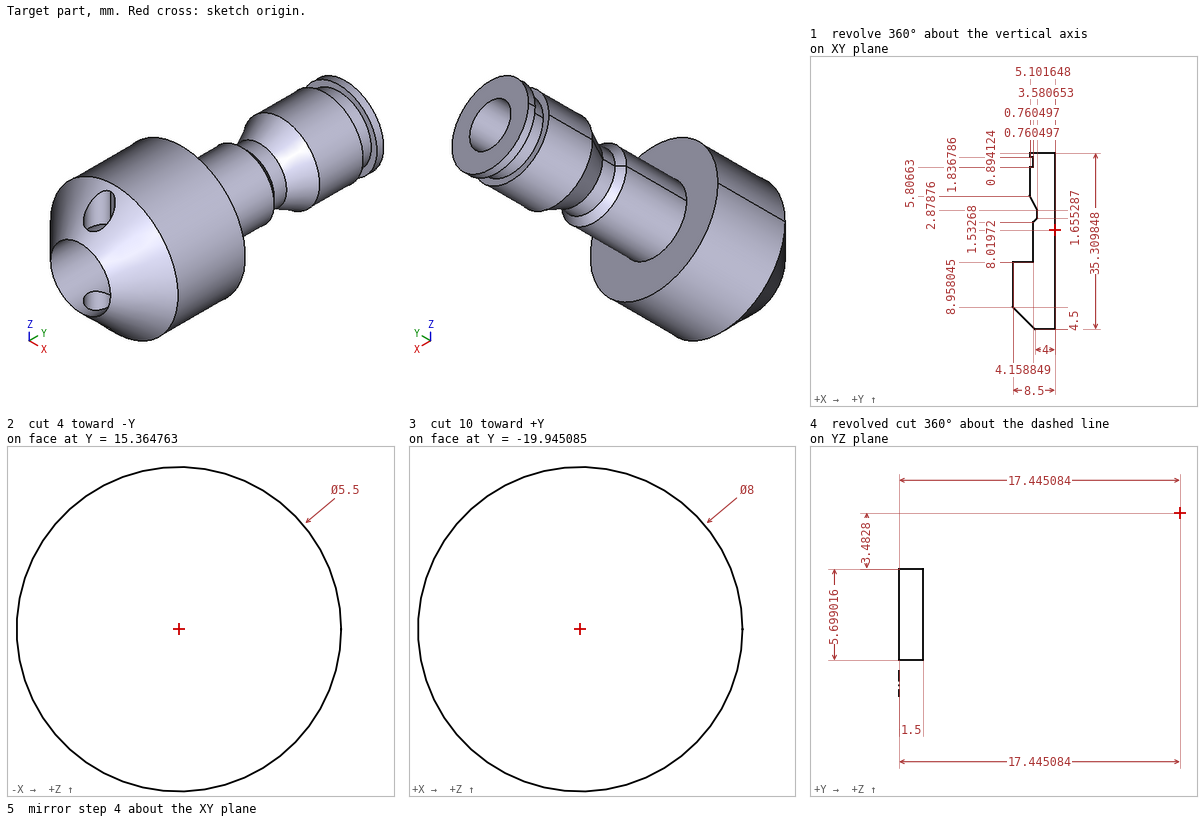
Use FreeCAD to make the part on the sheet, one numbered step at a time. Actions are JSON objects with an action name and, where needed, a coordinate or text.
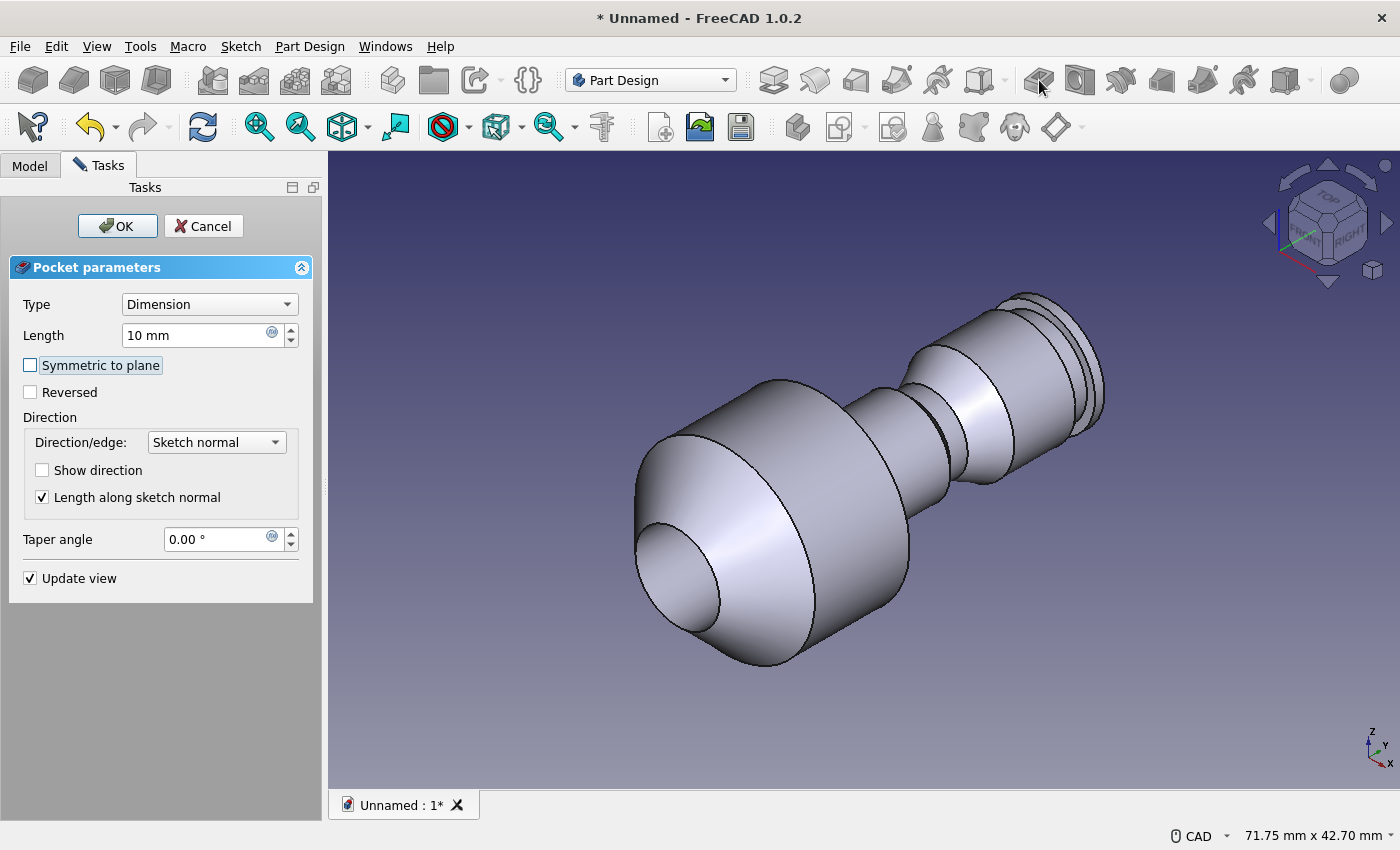
{"action": "left_click", "coordinate": [118, 226]}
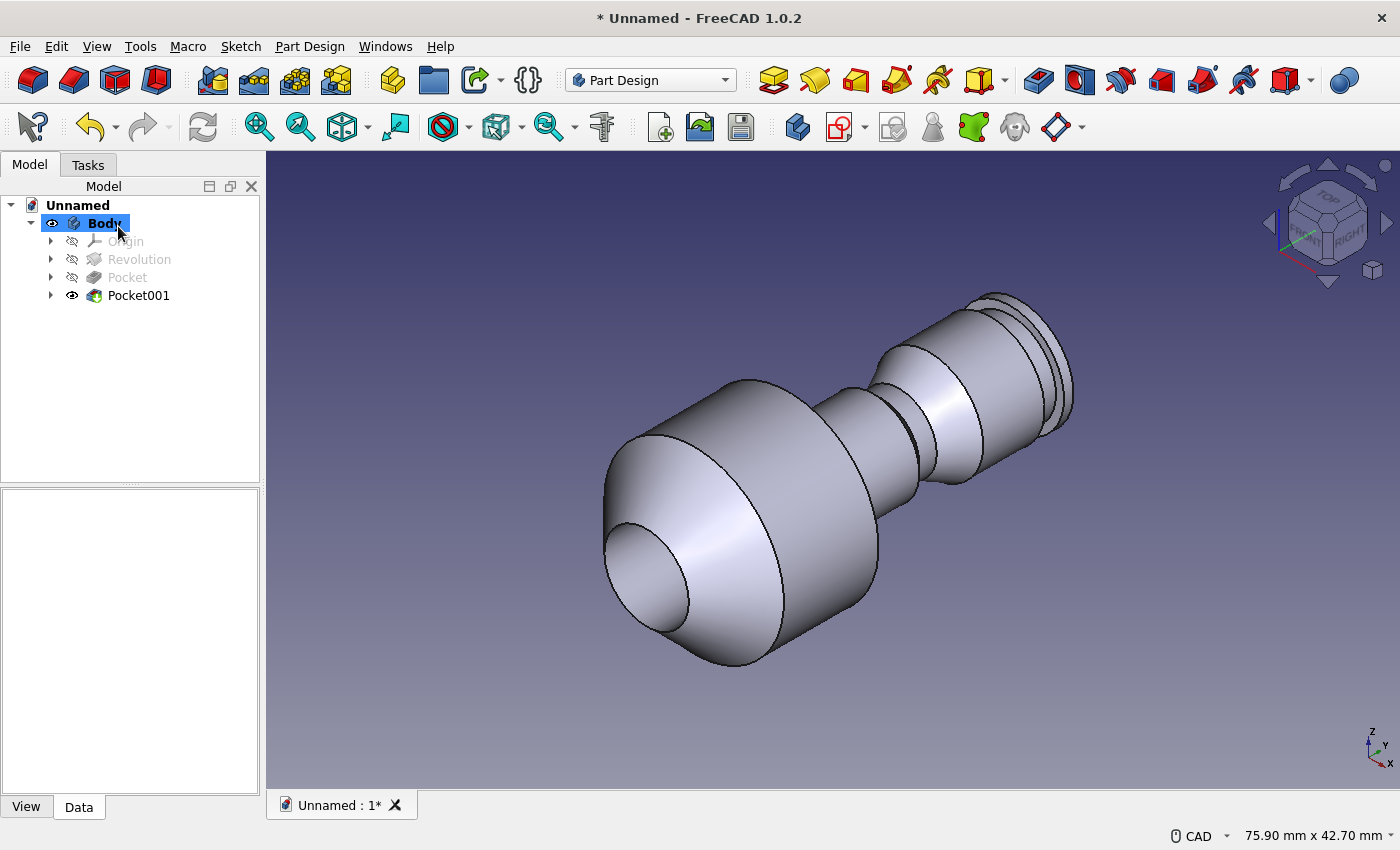
{"action": "left_click", "coordinate": [838, 128]}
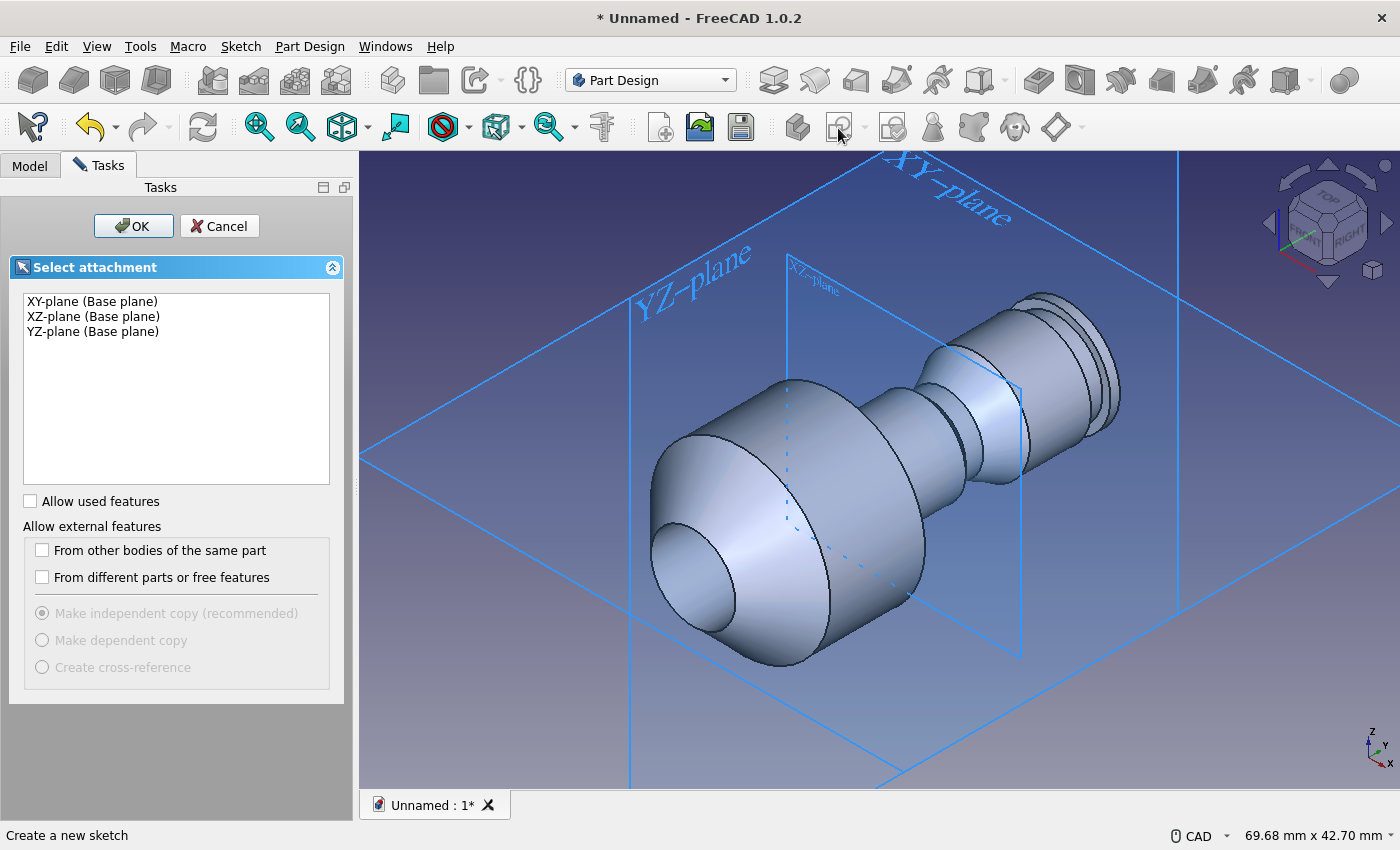
{"action": "left_click", "coordinate": [84, 332]}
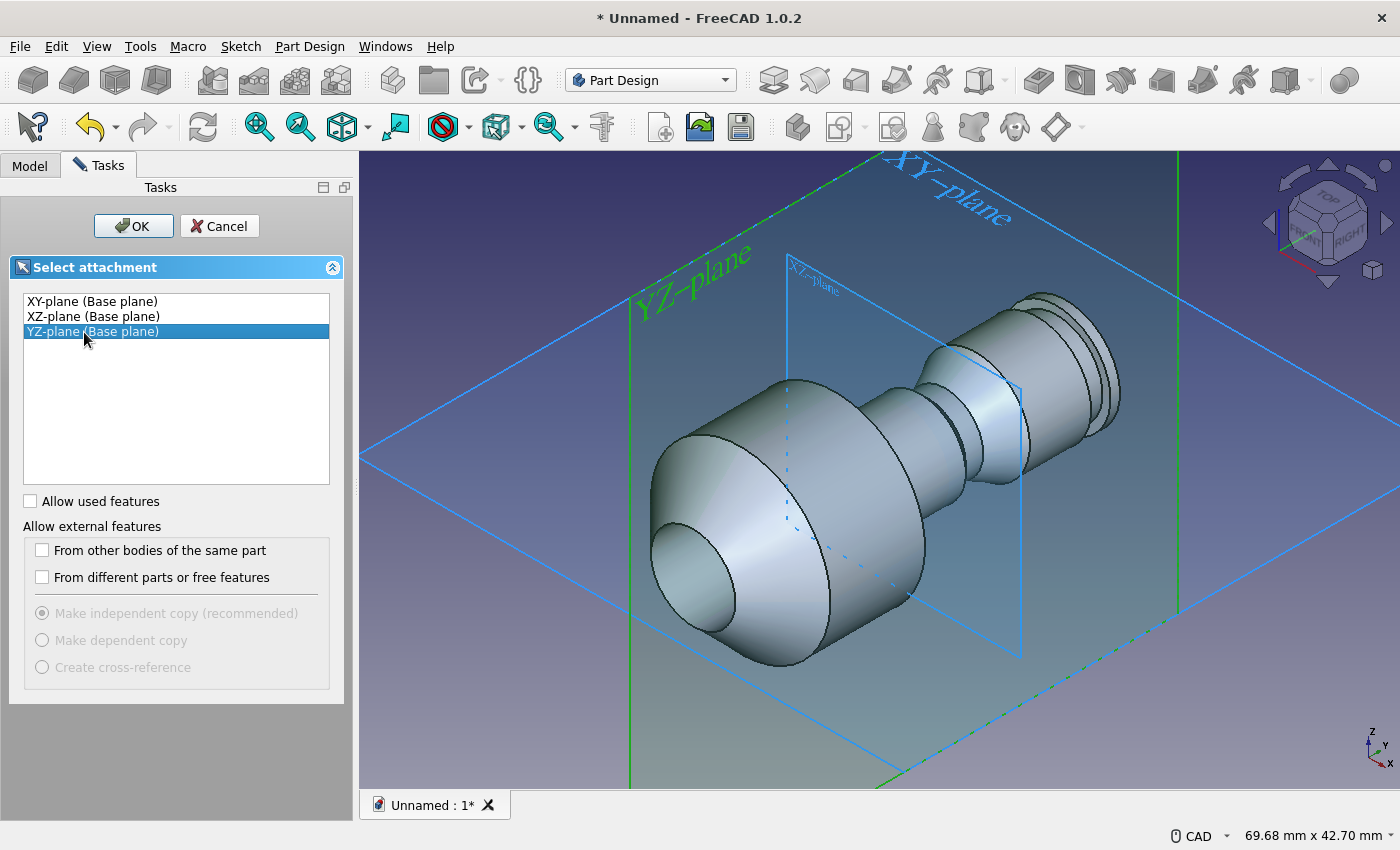
{"action": "left_click", "coordinate": [134, 226]}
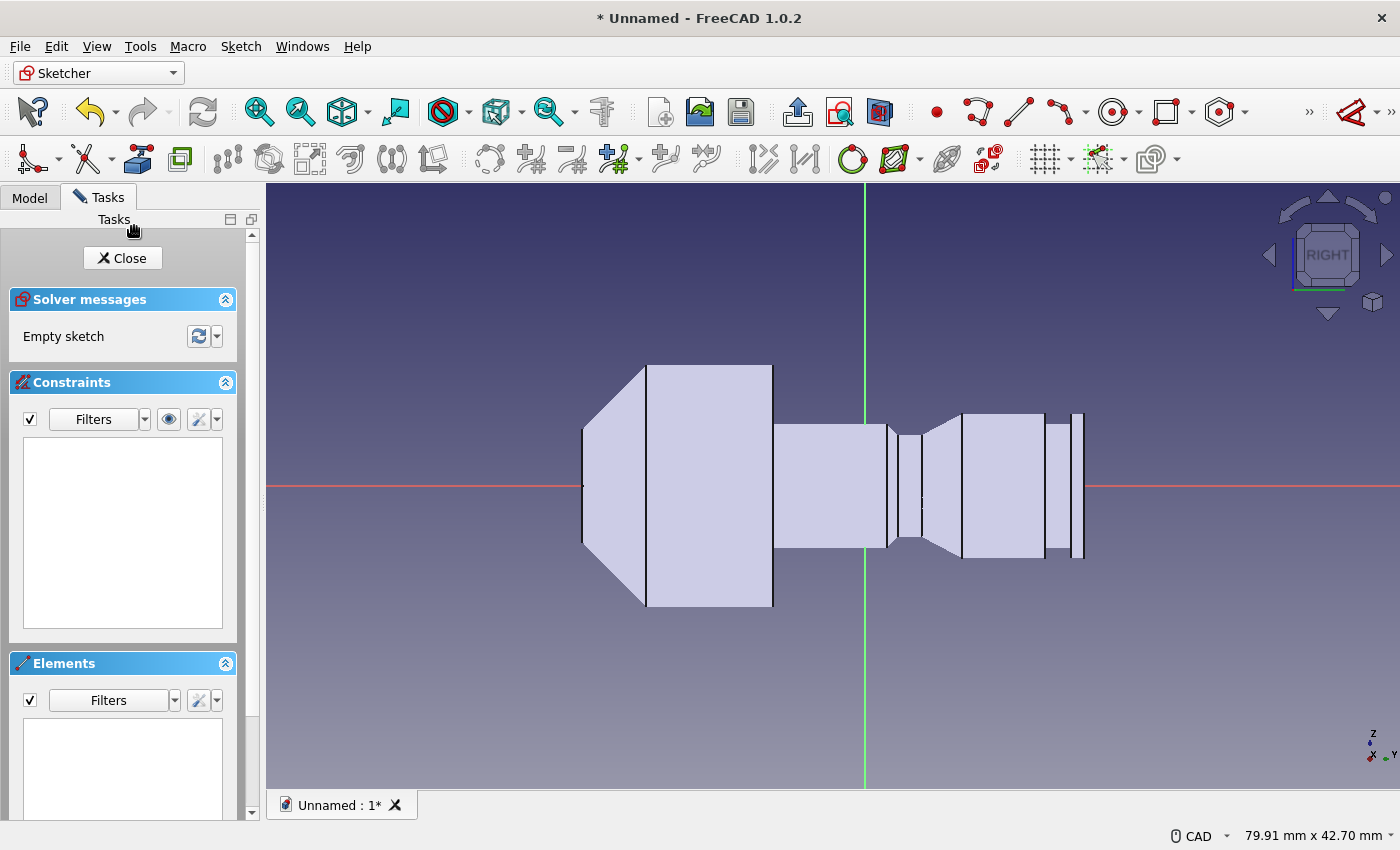
{"action": "left_click", "coordinate": [880, 112]}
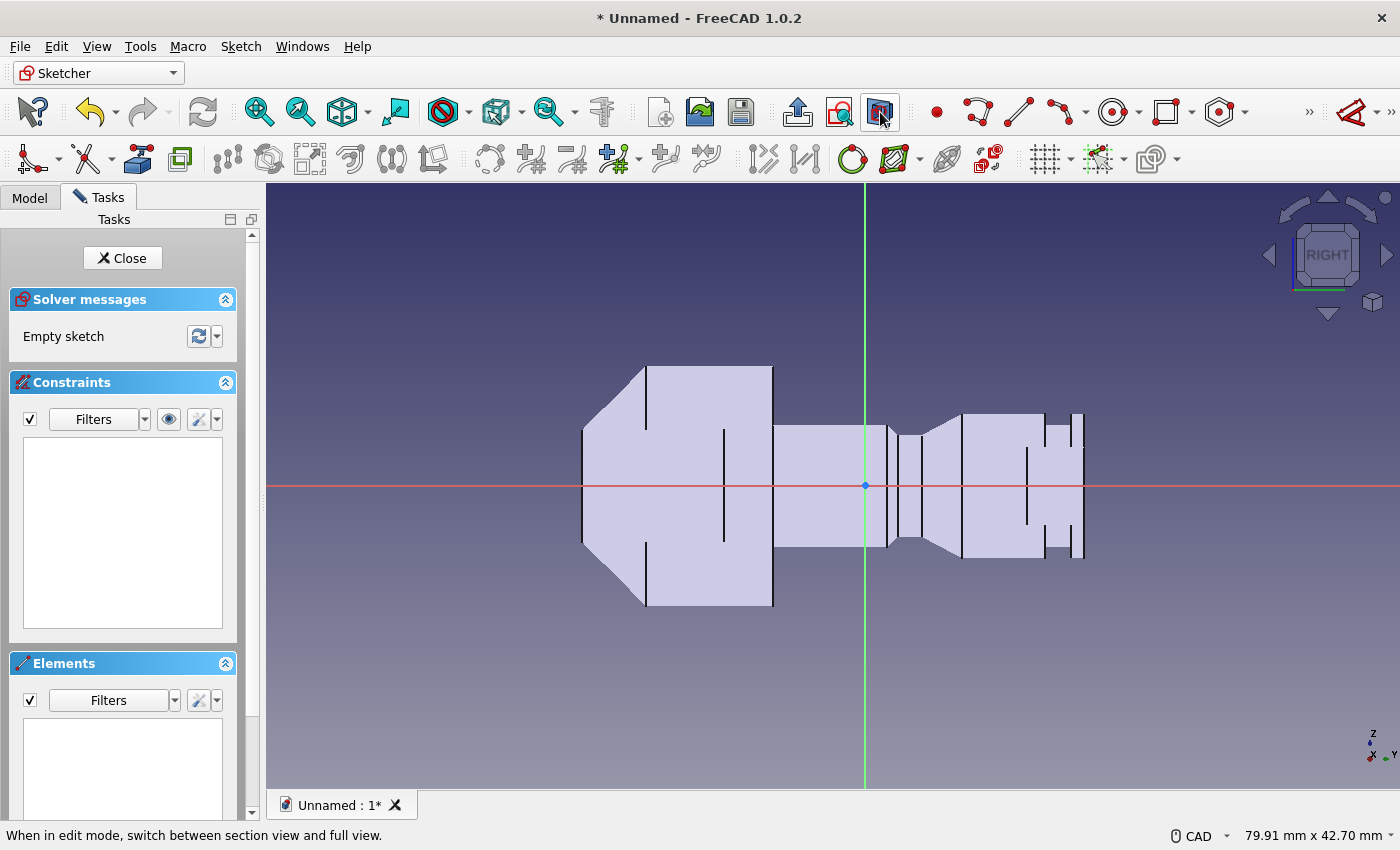
{"action": "scroll", "coordinate": [723, 634], "scroll_direction": "up", "scroll_amount": 4}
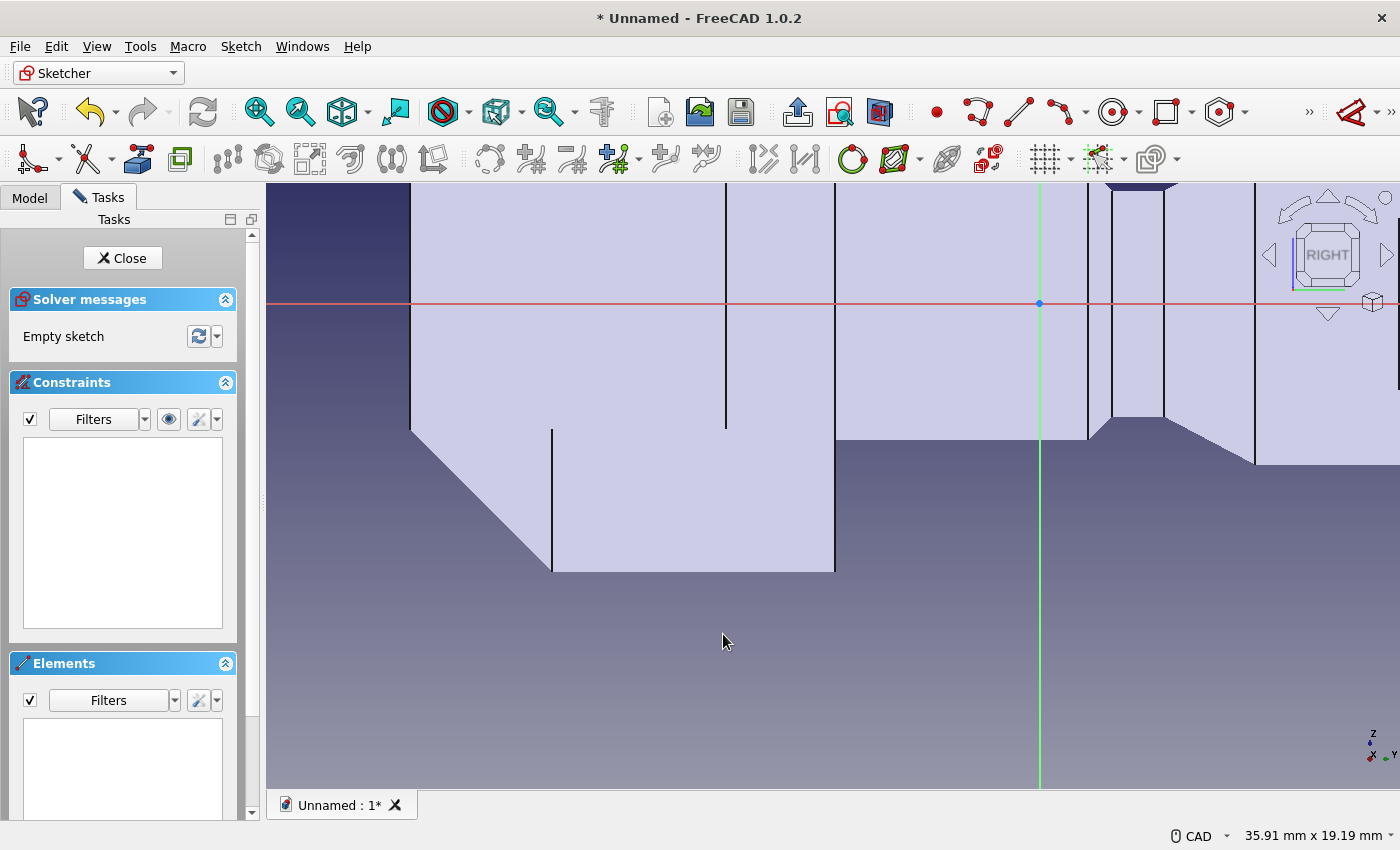
{"action": "left_click", "coordinate": [1166, 112]}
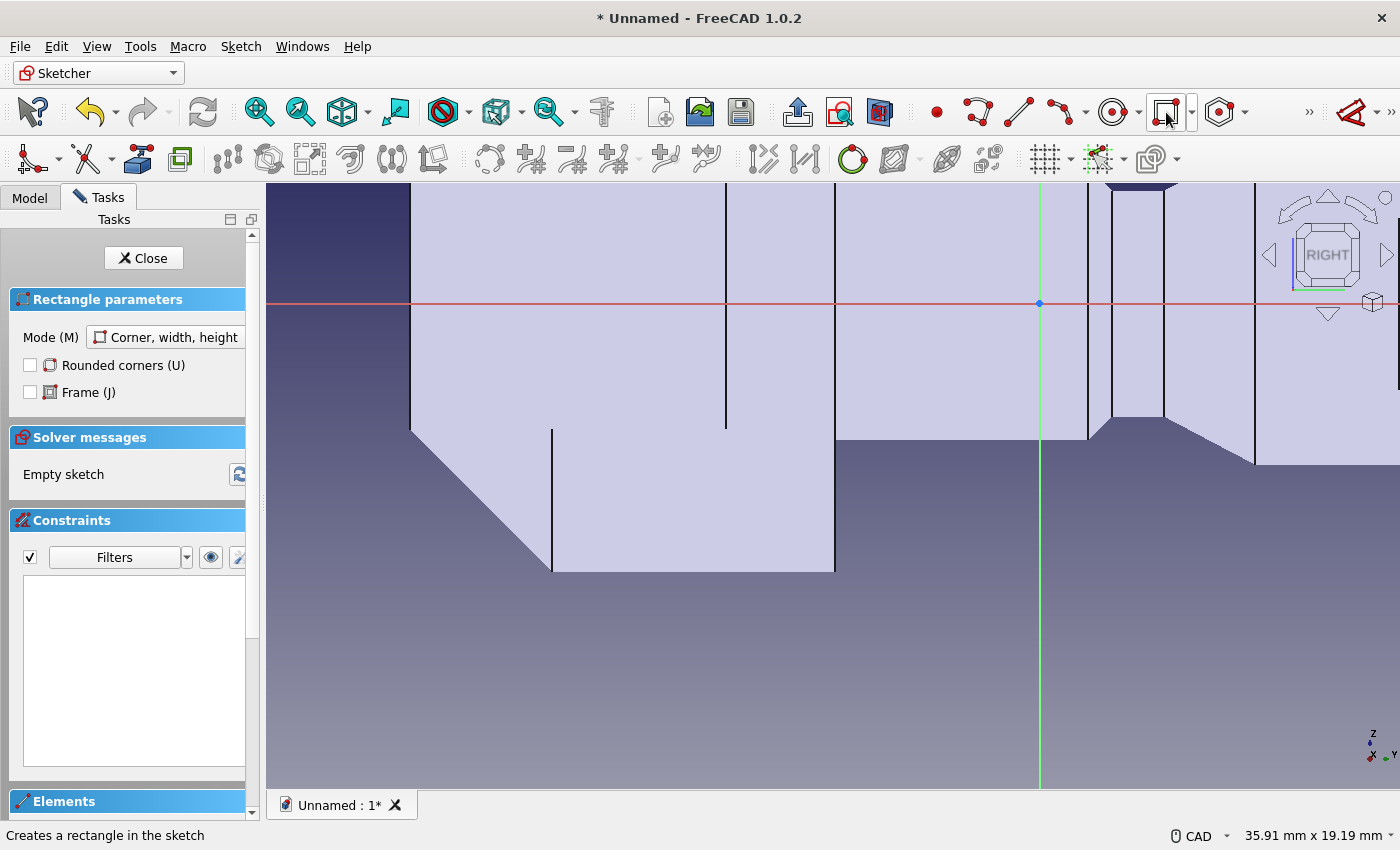
{"action": "left_click", "coordinate": [489, 414]}
{"action": "left_click", "coordinate": [536, 594]}